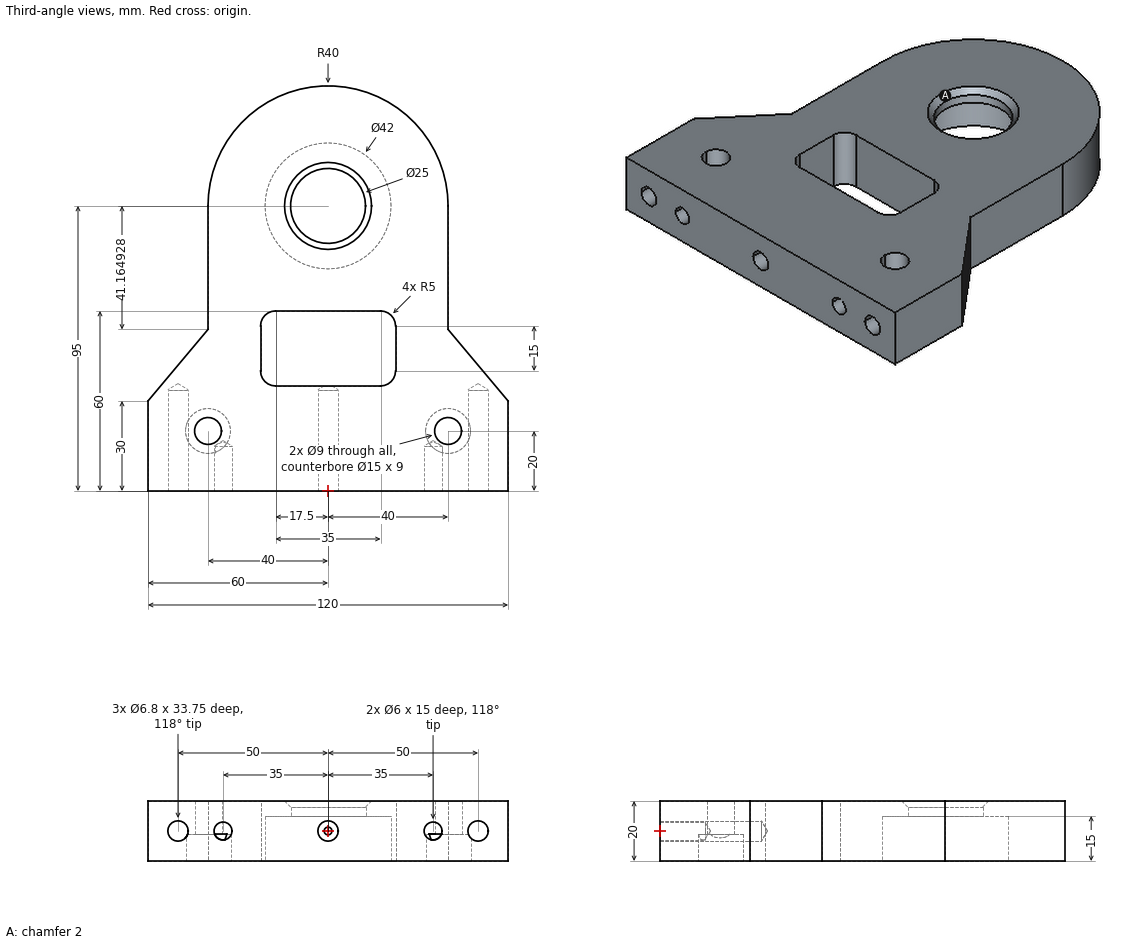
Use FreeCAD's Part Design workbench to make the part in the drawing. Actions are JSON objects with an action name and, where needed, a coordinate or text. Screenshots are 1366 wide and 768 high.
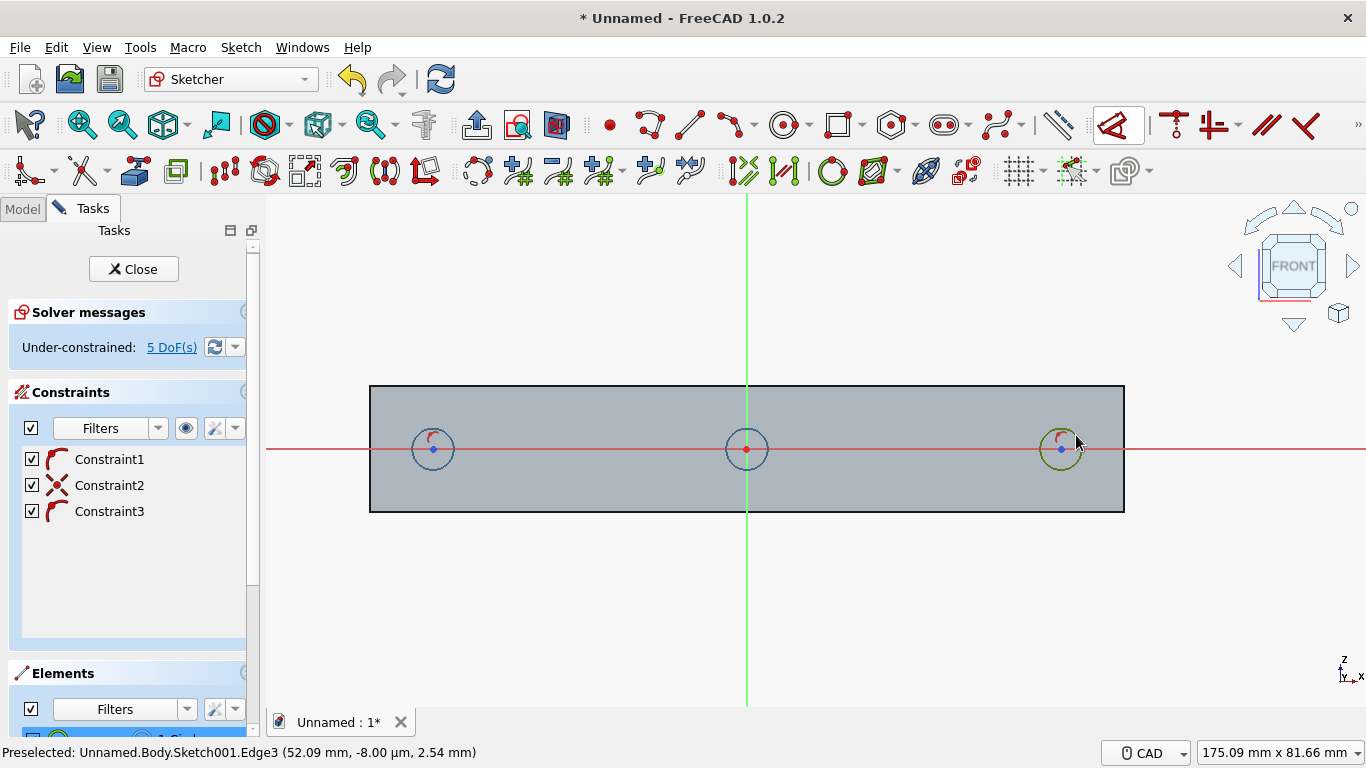
{"action": "key", "text": "e"}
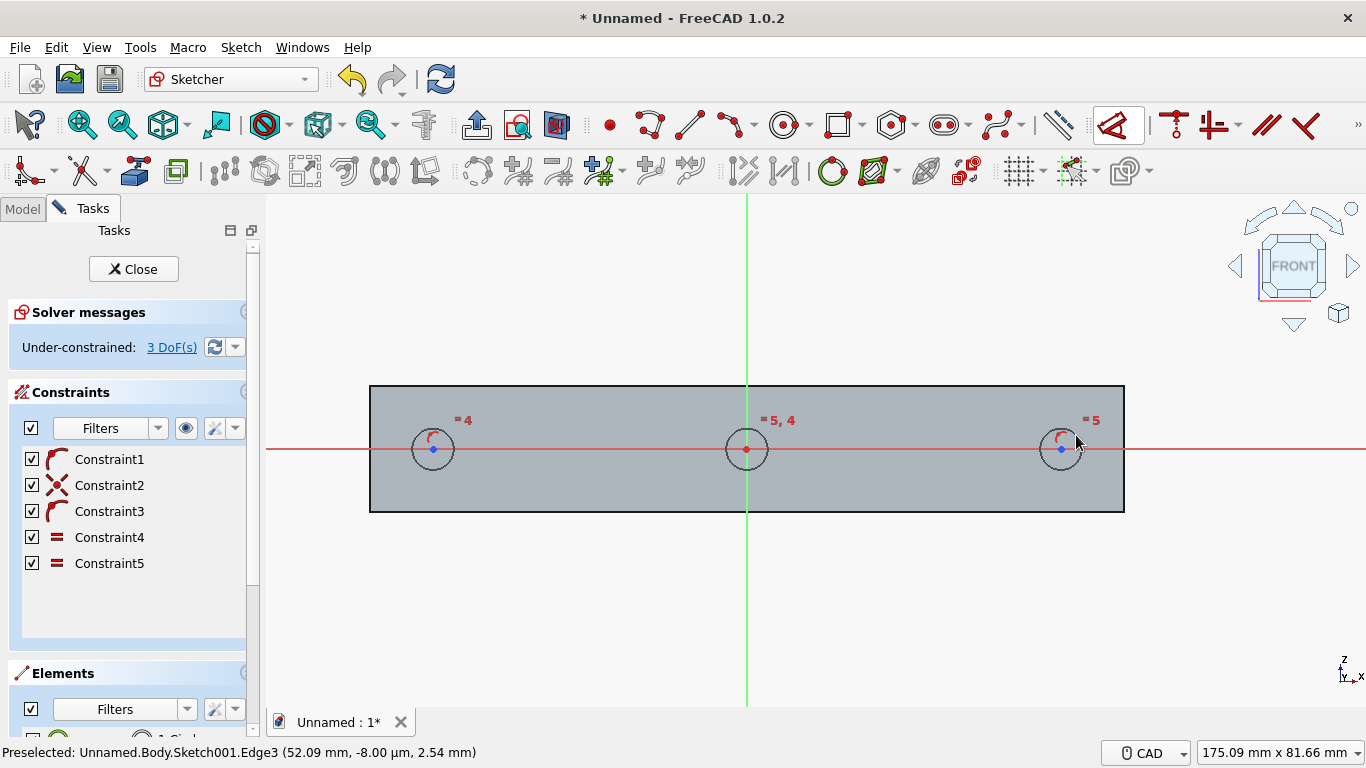
{"action": "left_click", "coordinate": [448, 435]}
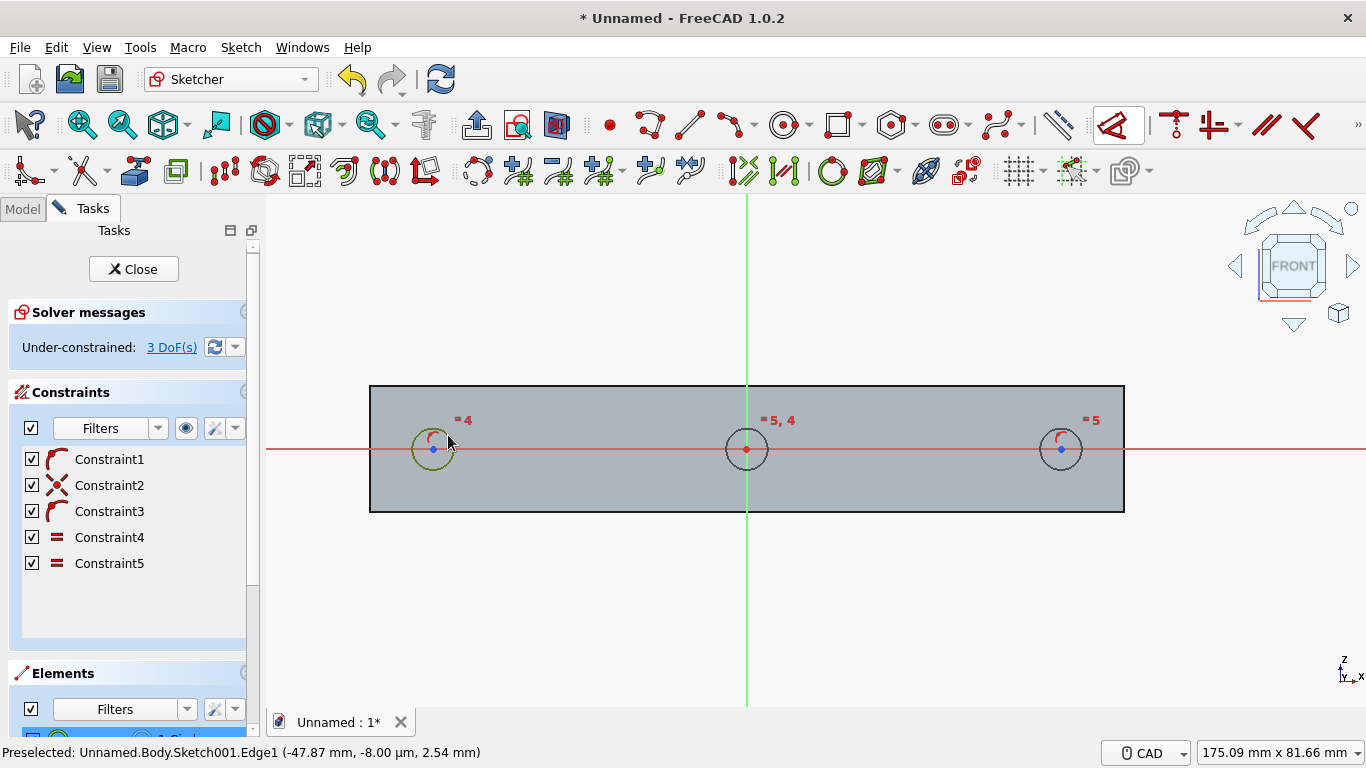
{"action": "key", "text": "k o"}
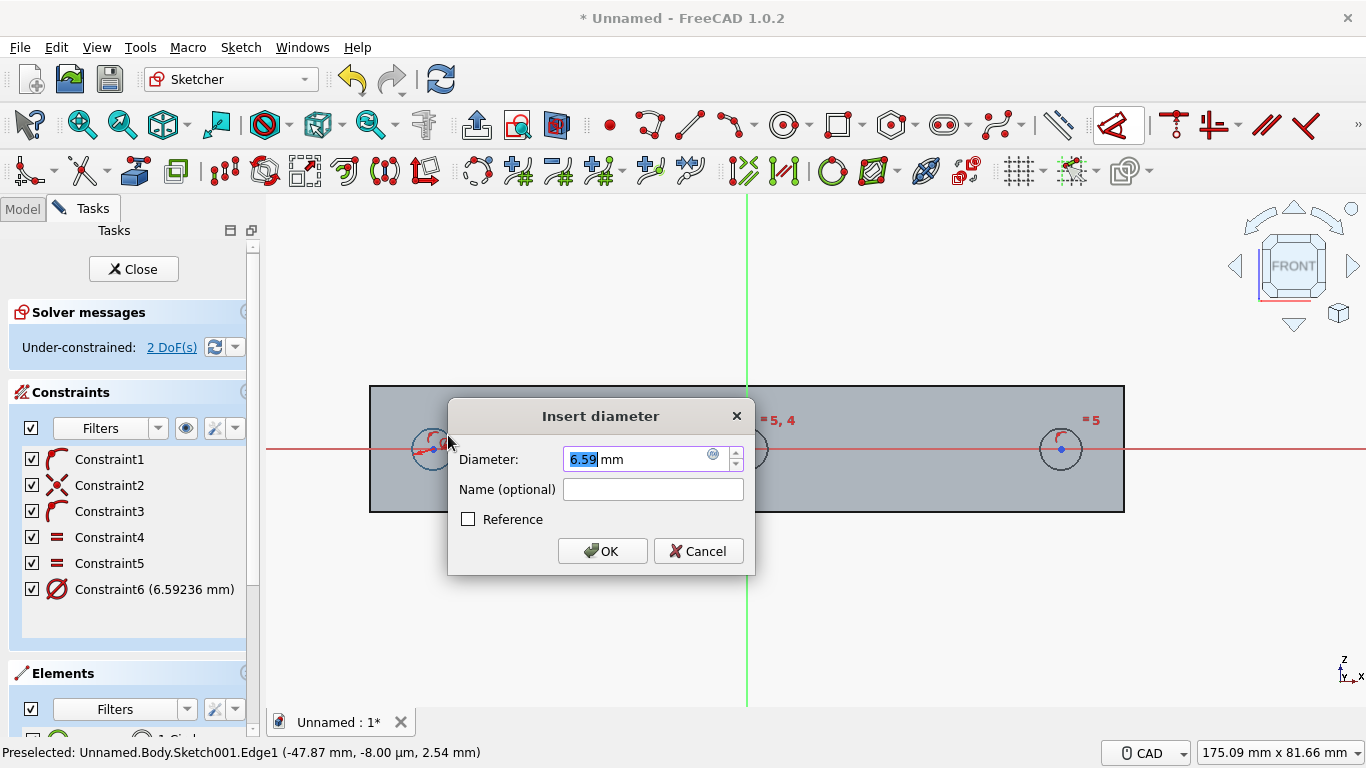
{"action": "type", "text": "6.8"}
{"action": "key", "text": "Return"}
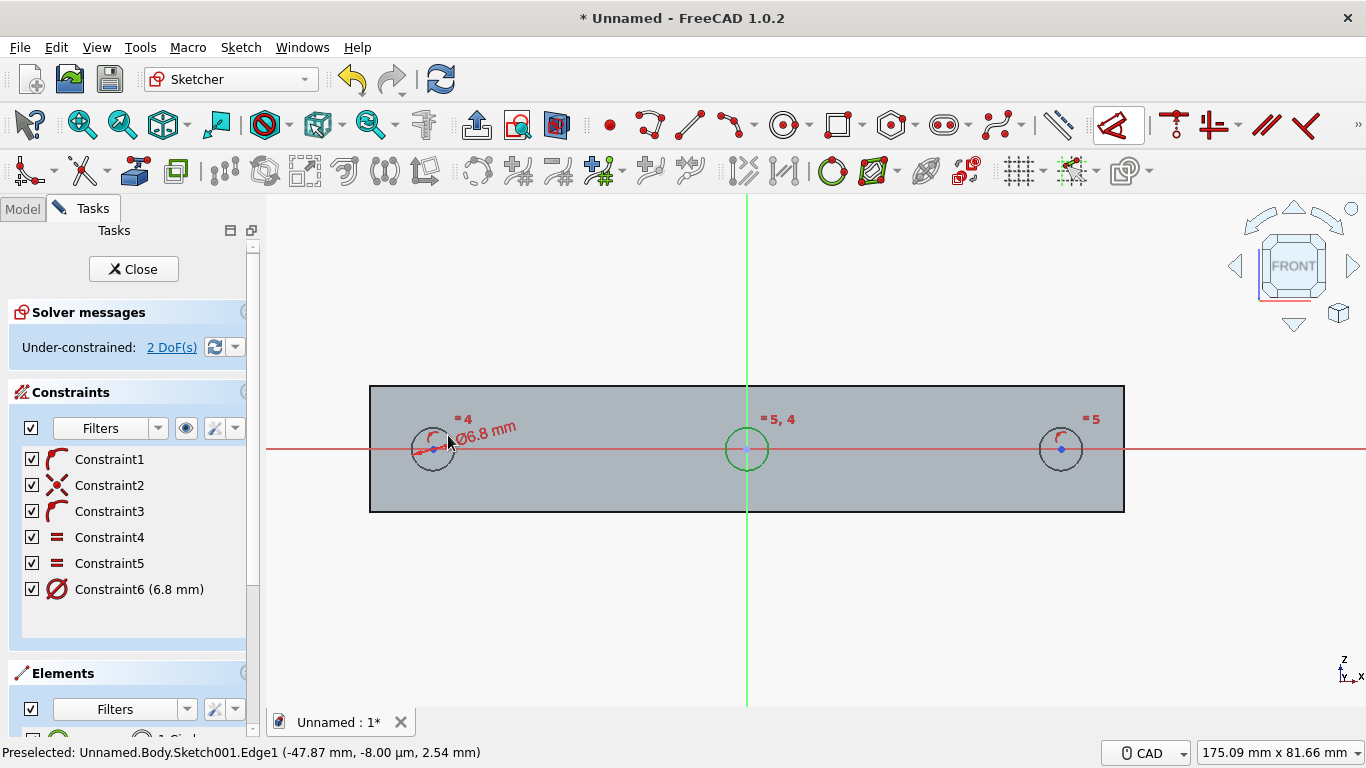
{"action": "left_click", "coordinate": [433, 449]}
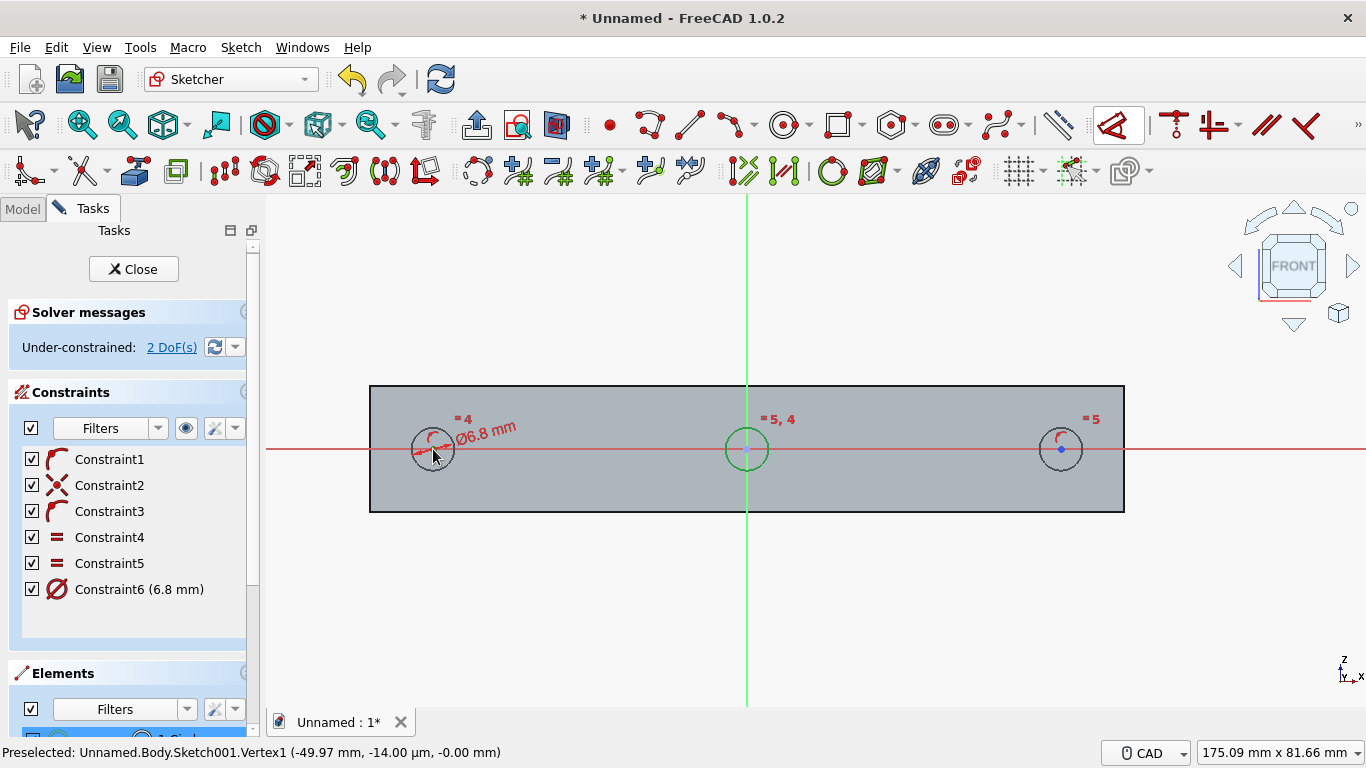
{"action": "key", "text": "l"}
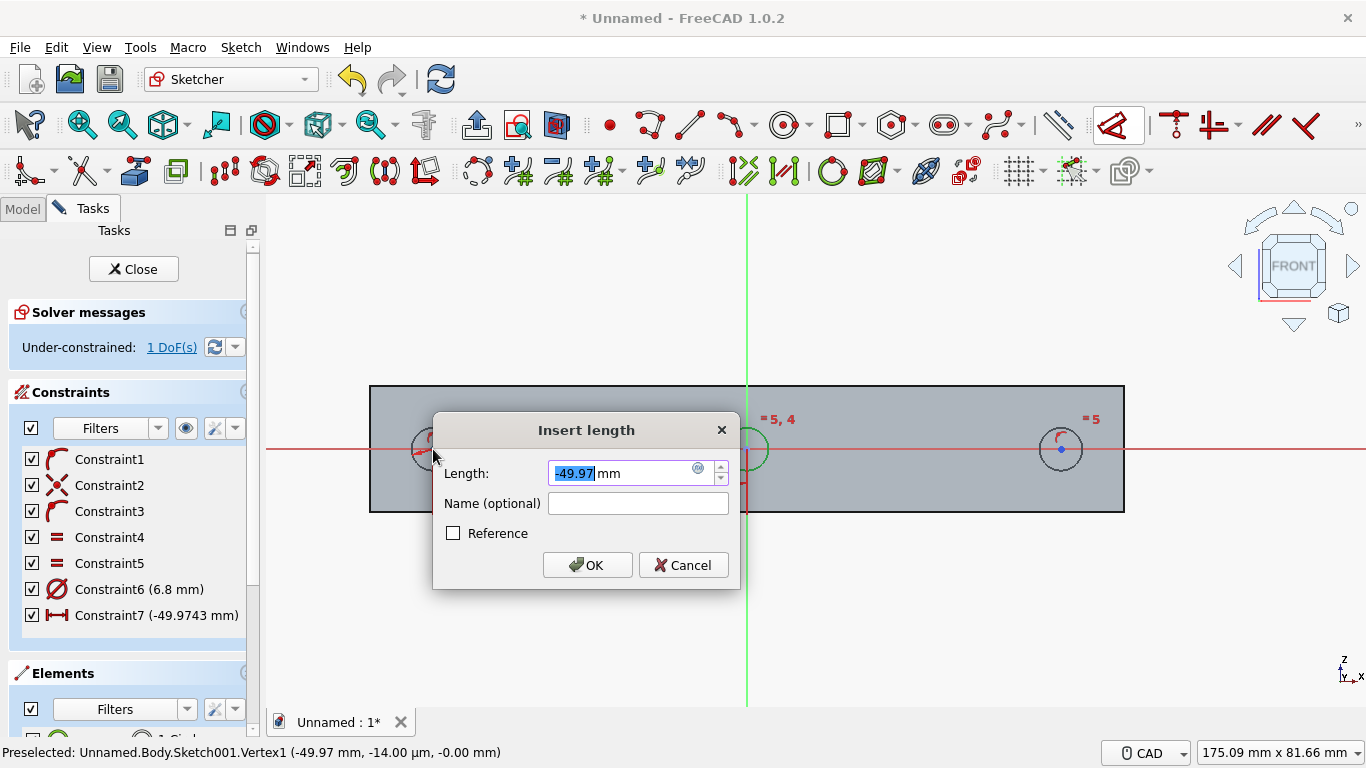
{"action": "type", "text": "-50"}
{"action": "key", "text": "Return"}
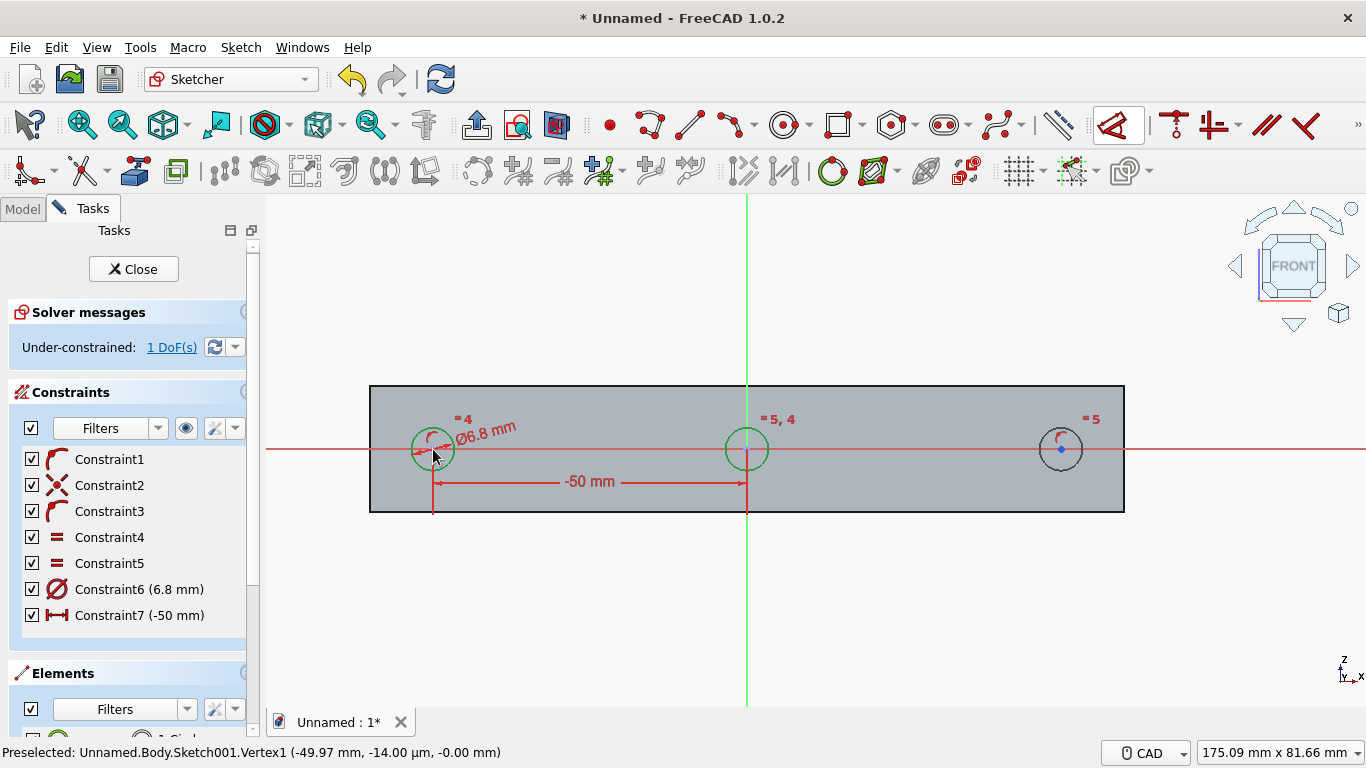
{"action": "left_click", "coordinate": [1061, 449]}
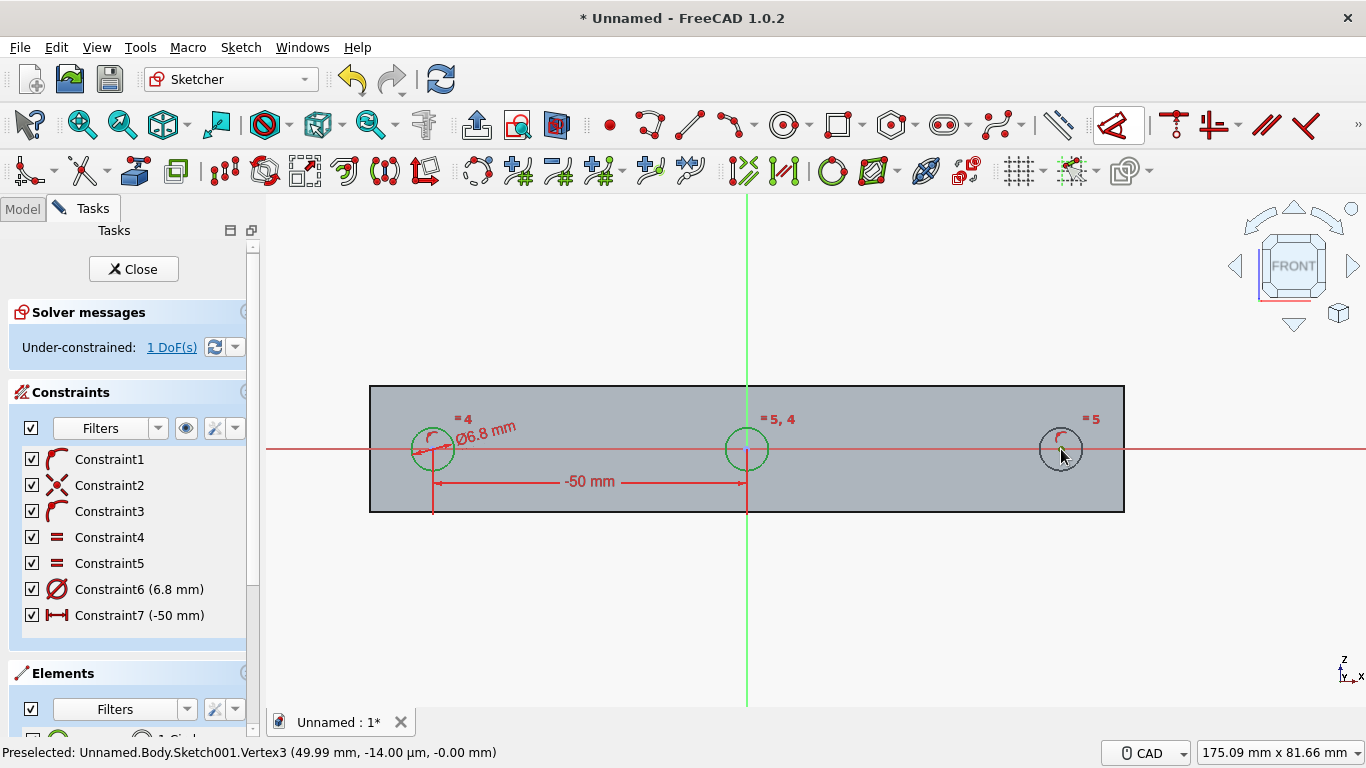
{"action": "key", "text": "l"}